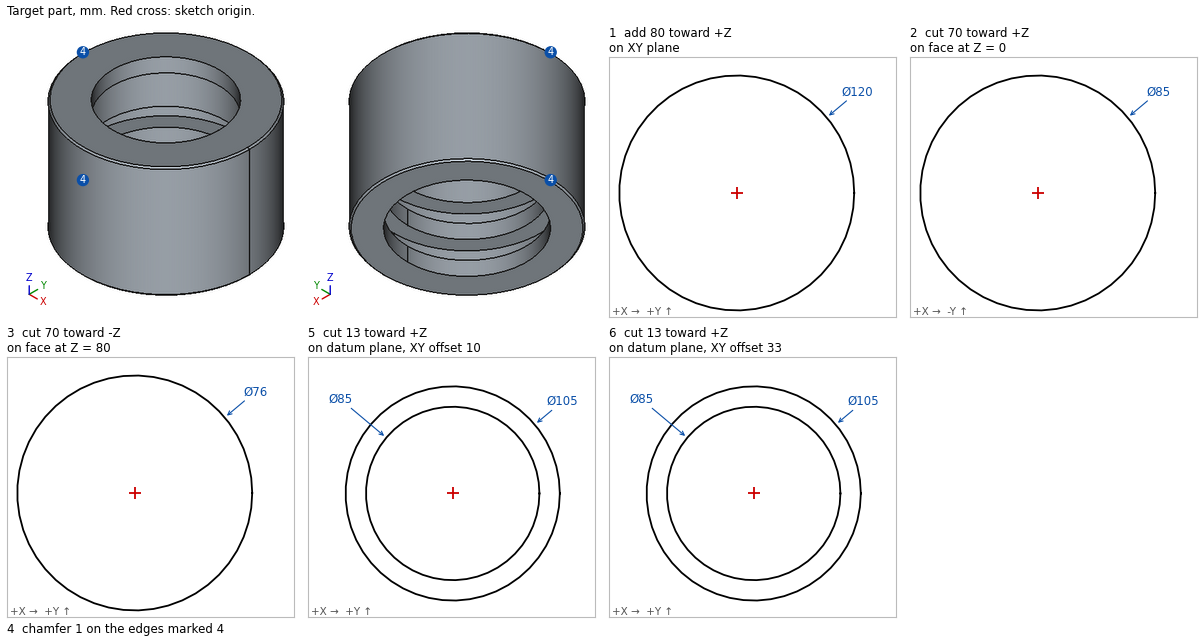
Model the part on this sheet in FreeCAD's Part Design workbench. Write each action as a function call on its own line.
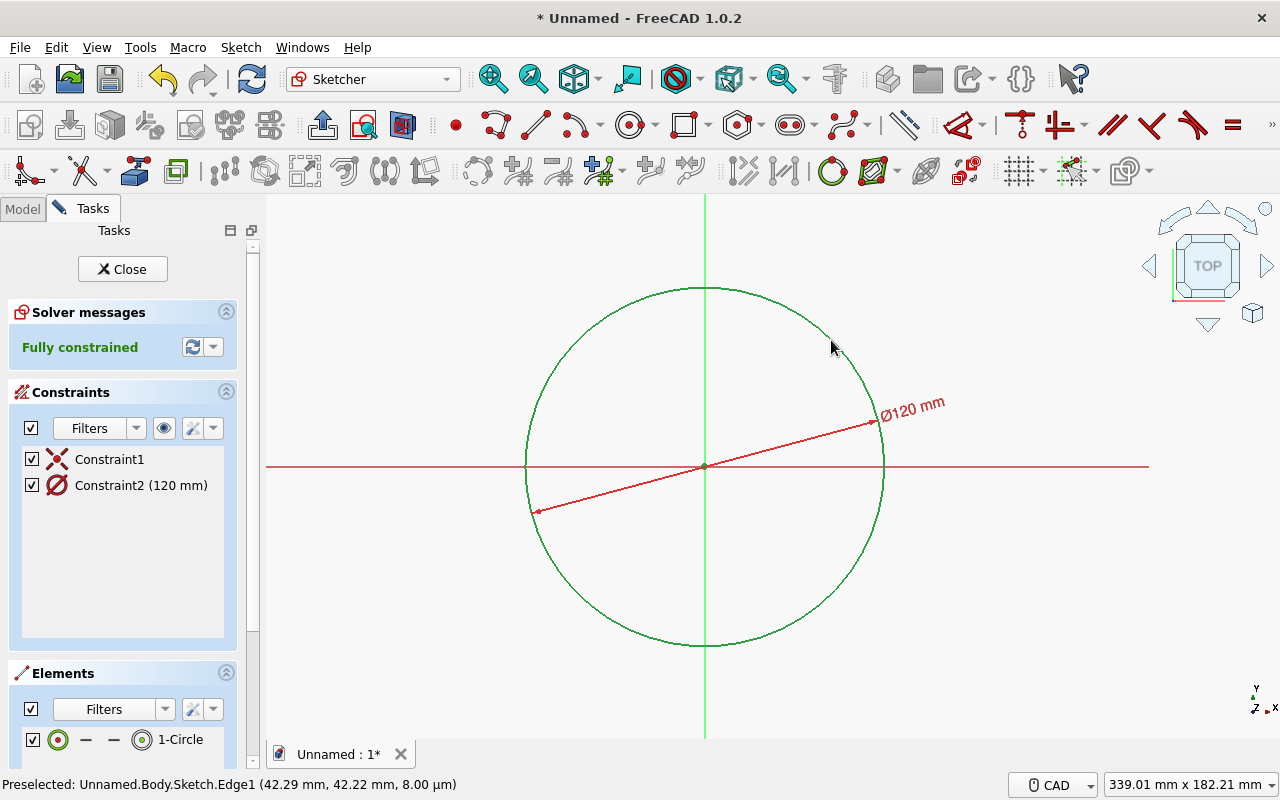
click(123, 269)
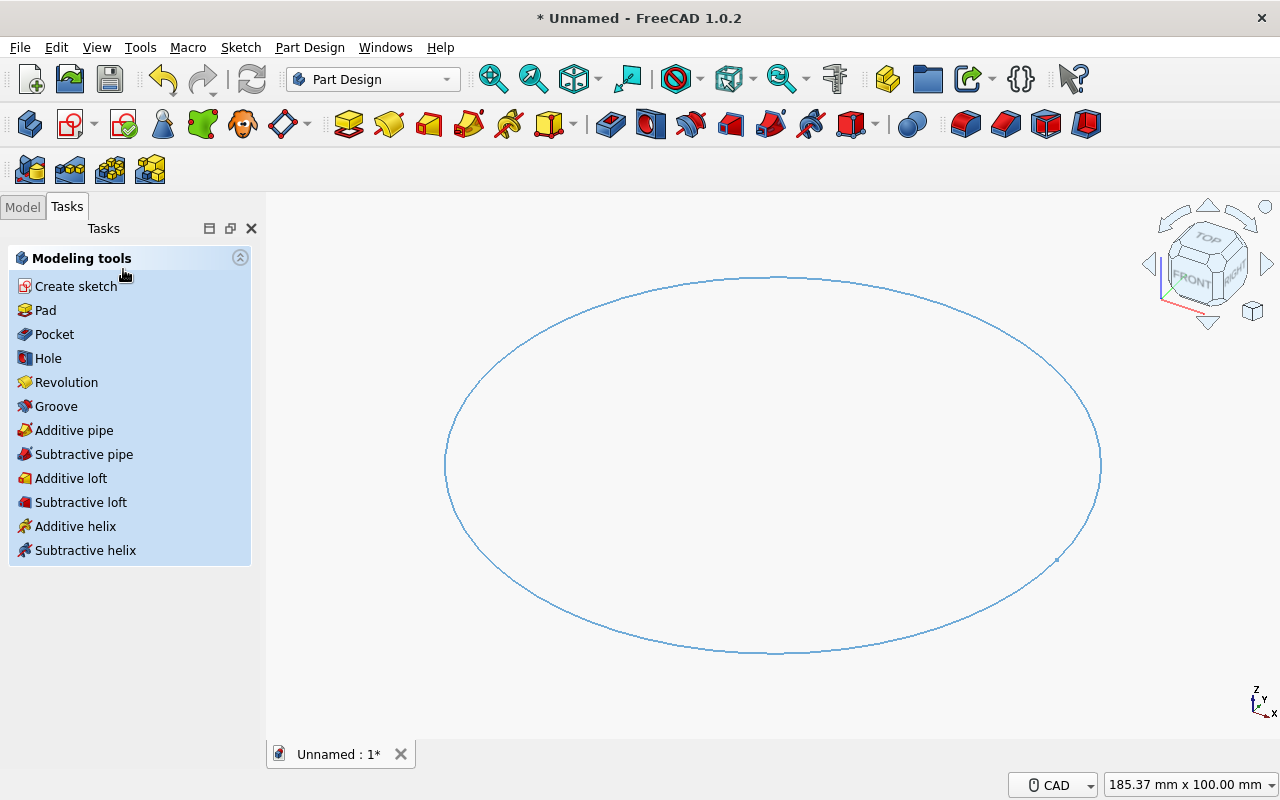
click(350, 124)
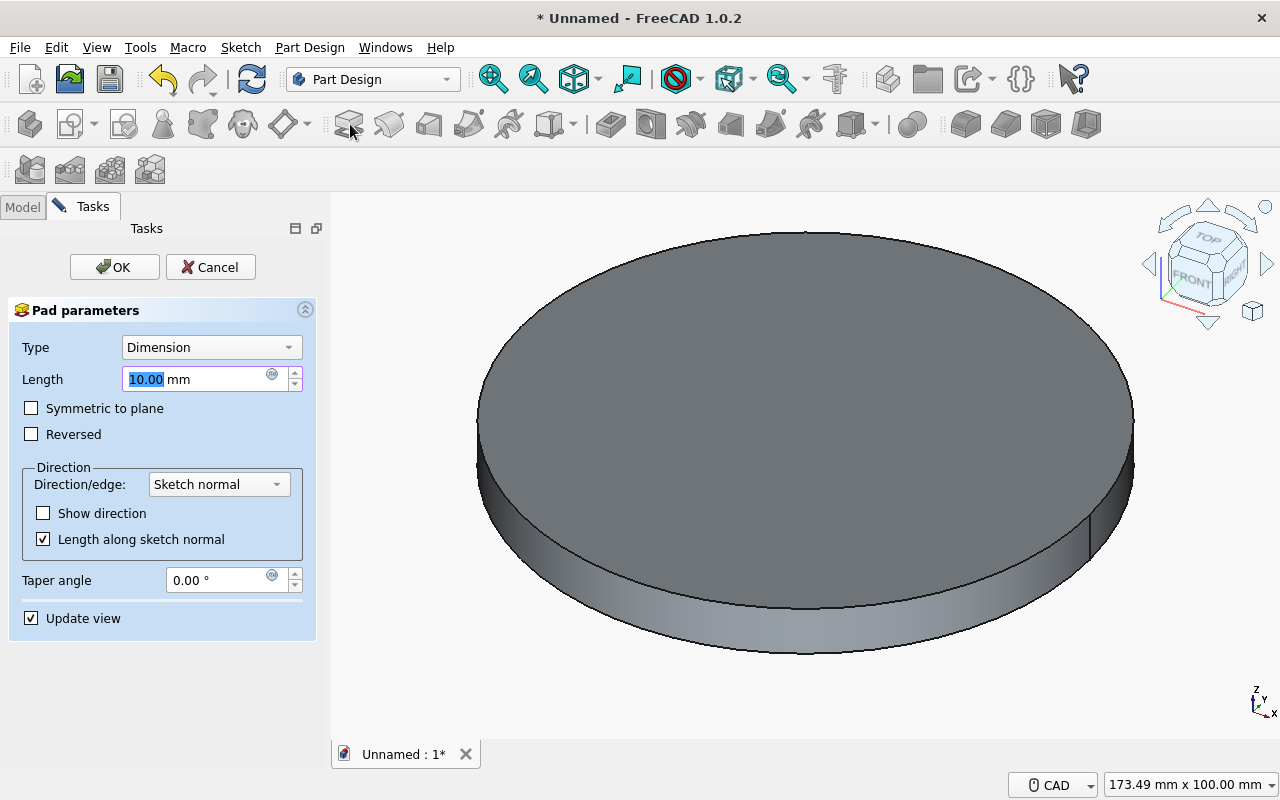
text(80)
key(Tab)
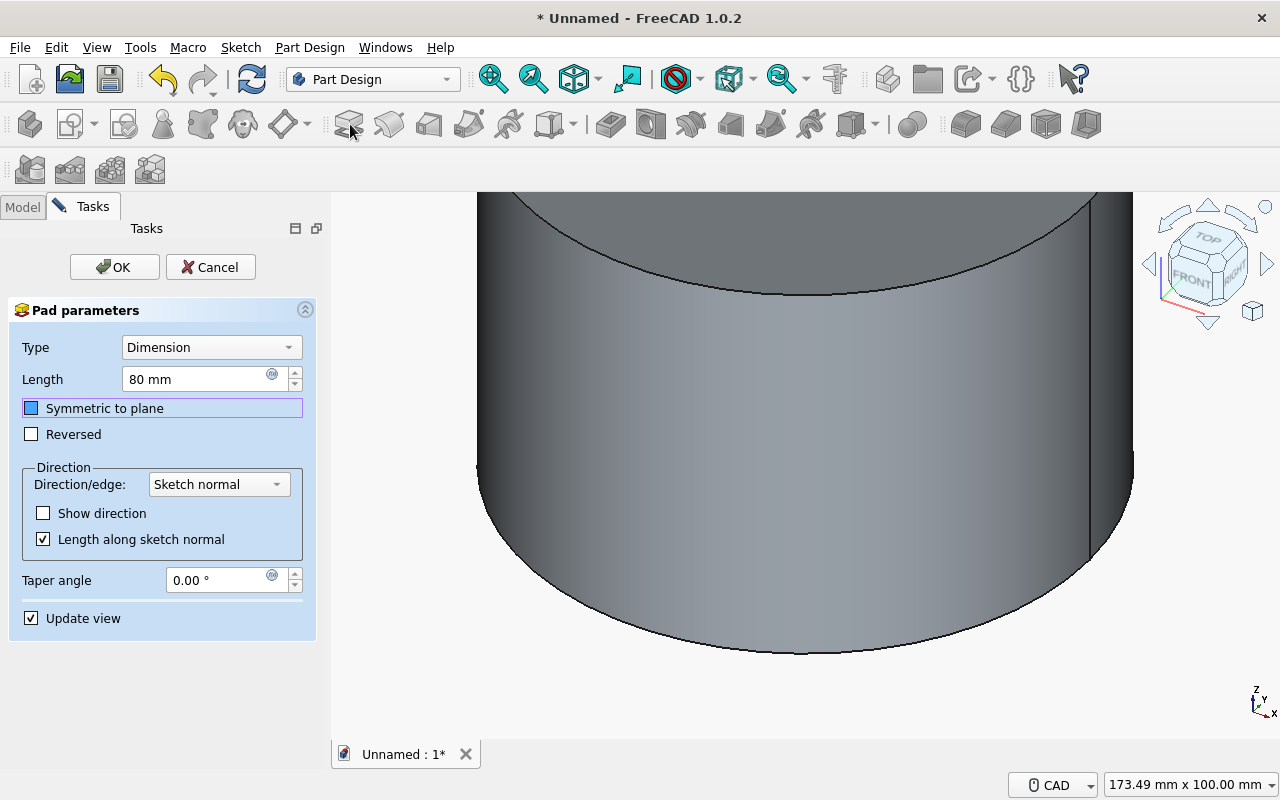
click(115, 267)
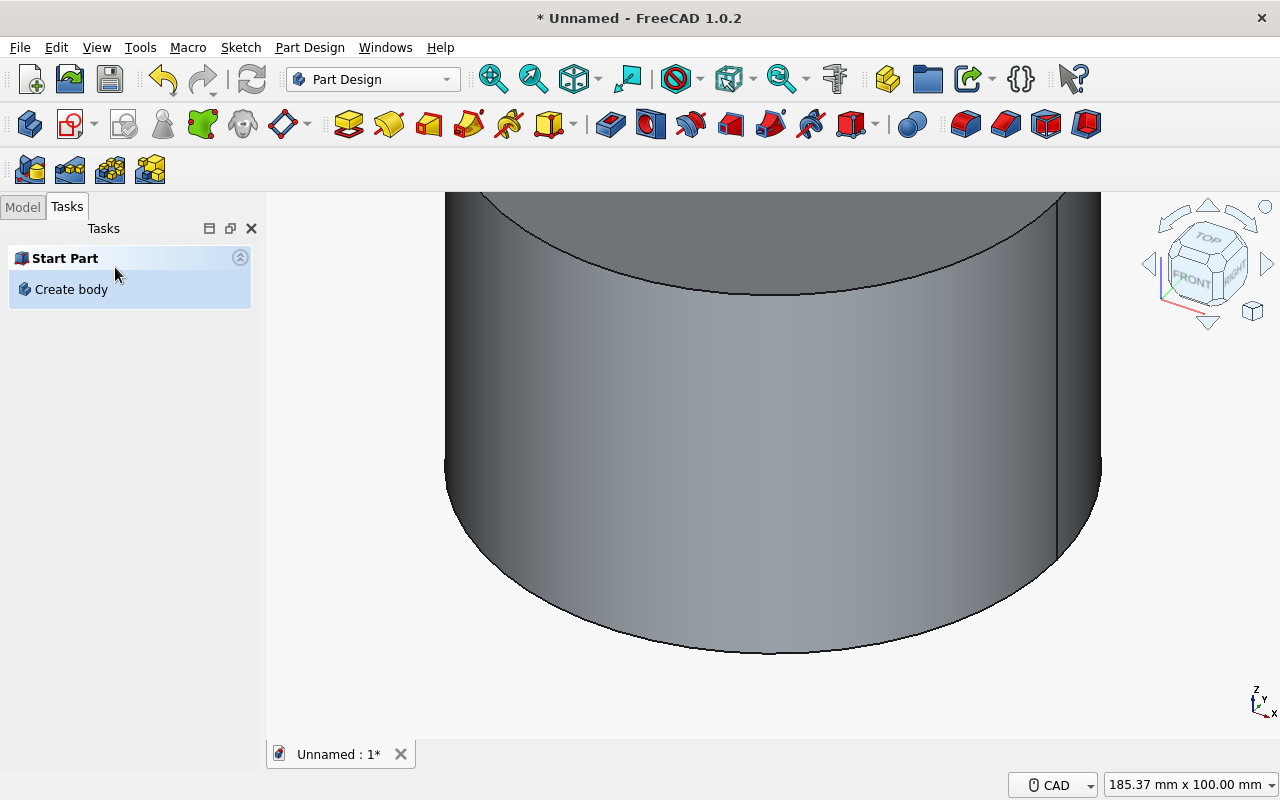
click(494, 80)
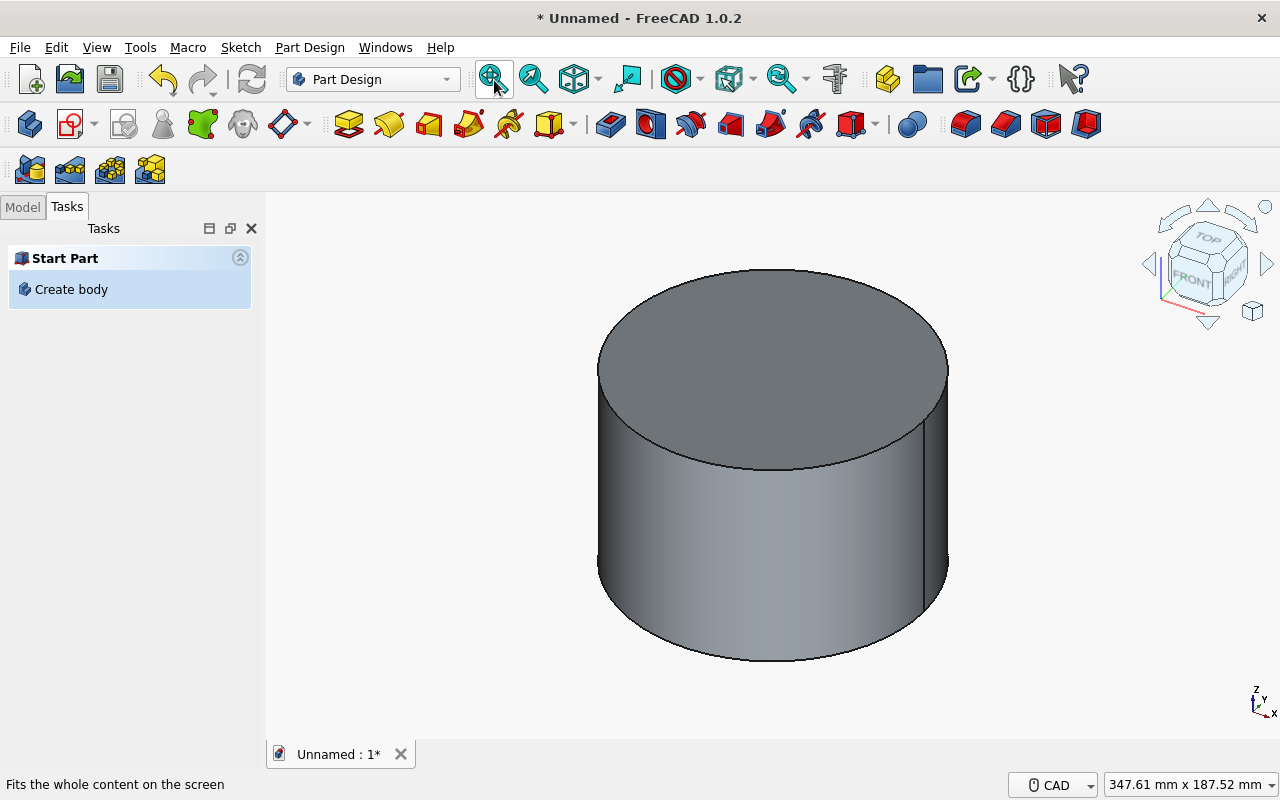
key(5)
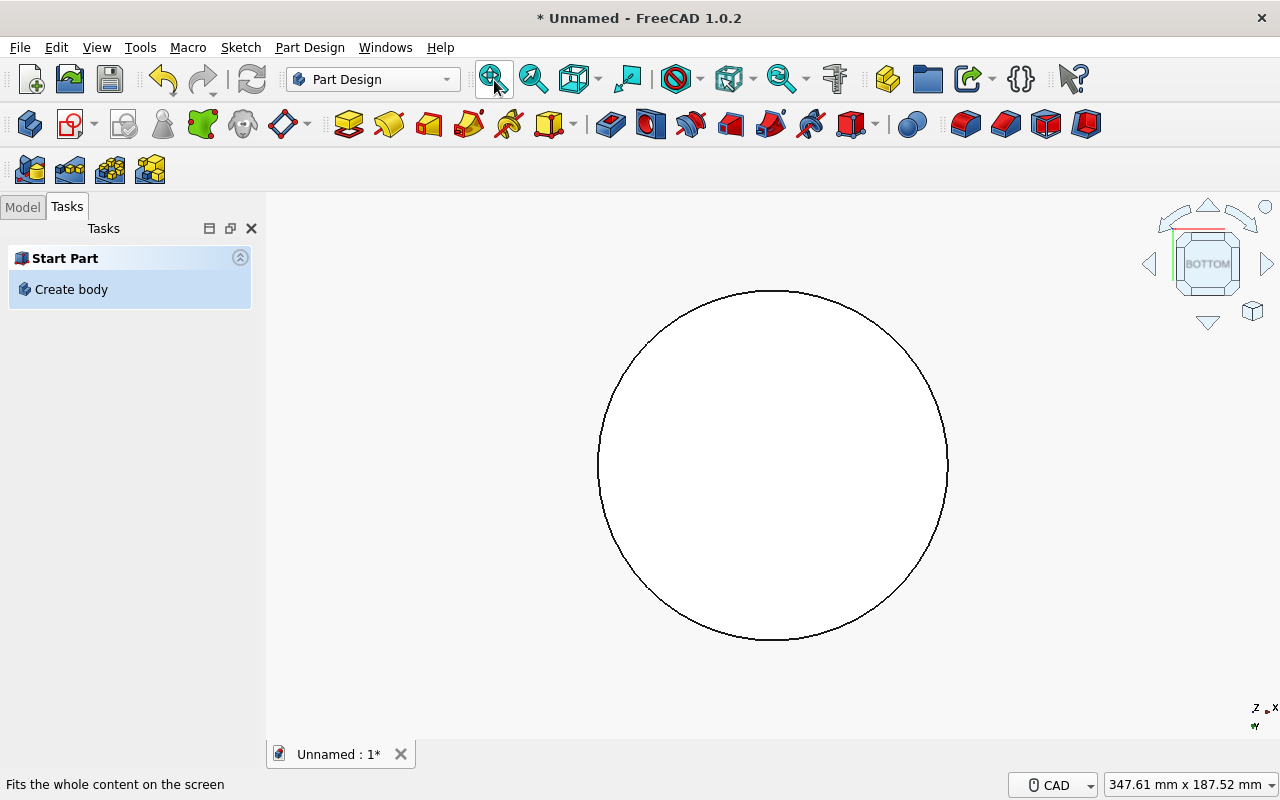
click(773, 464)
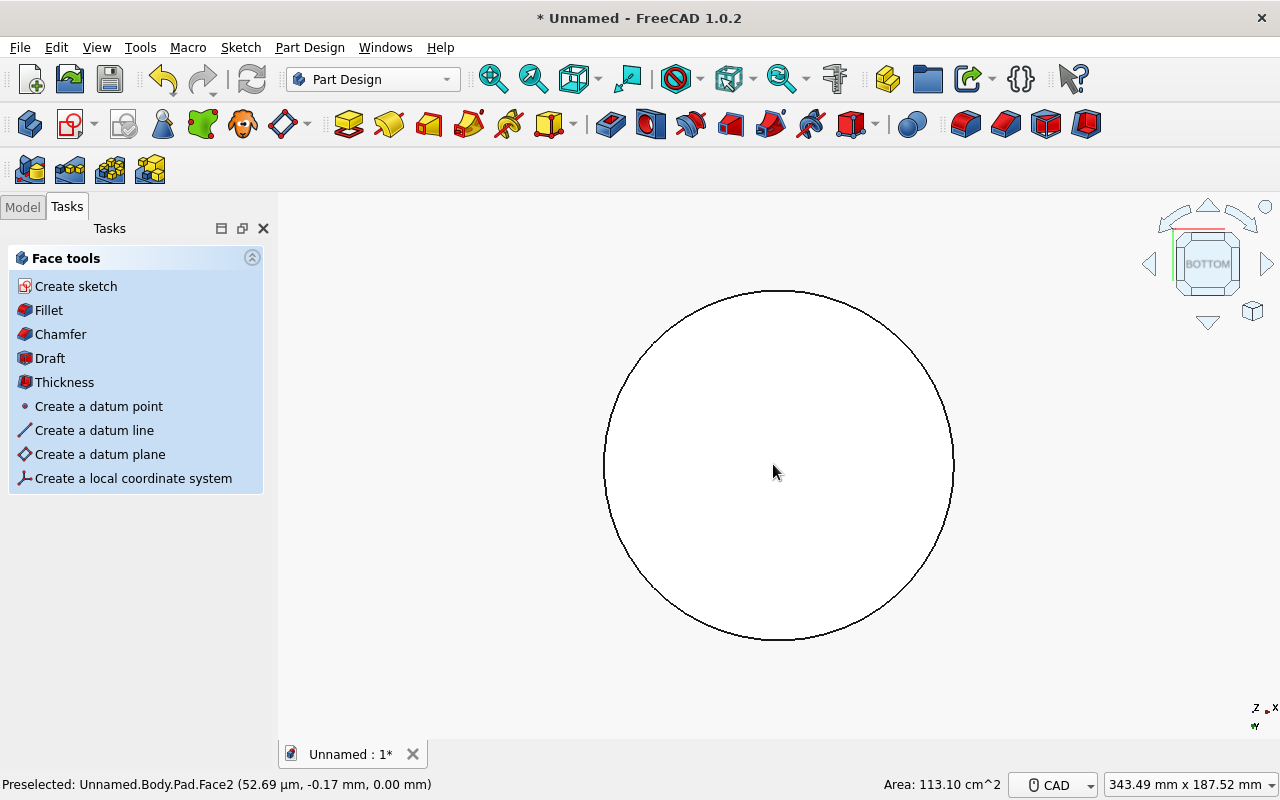
click(70, 124)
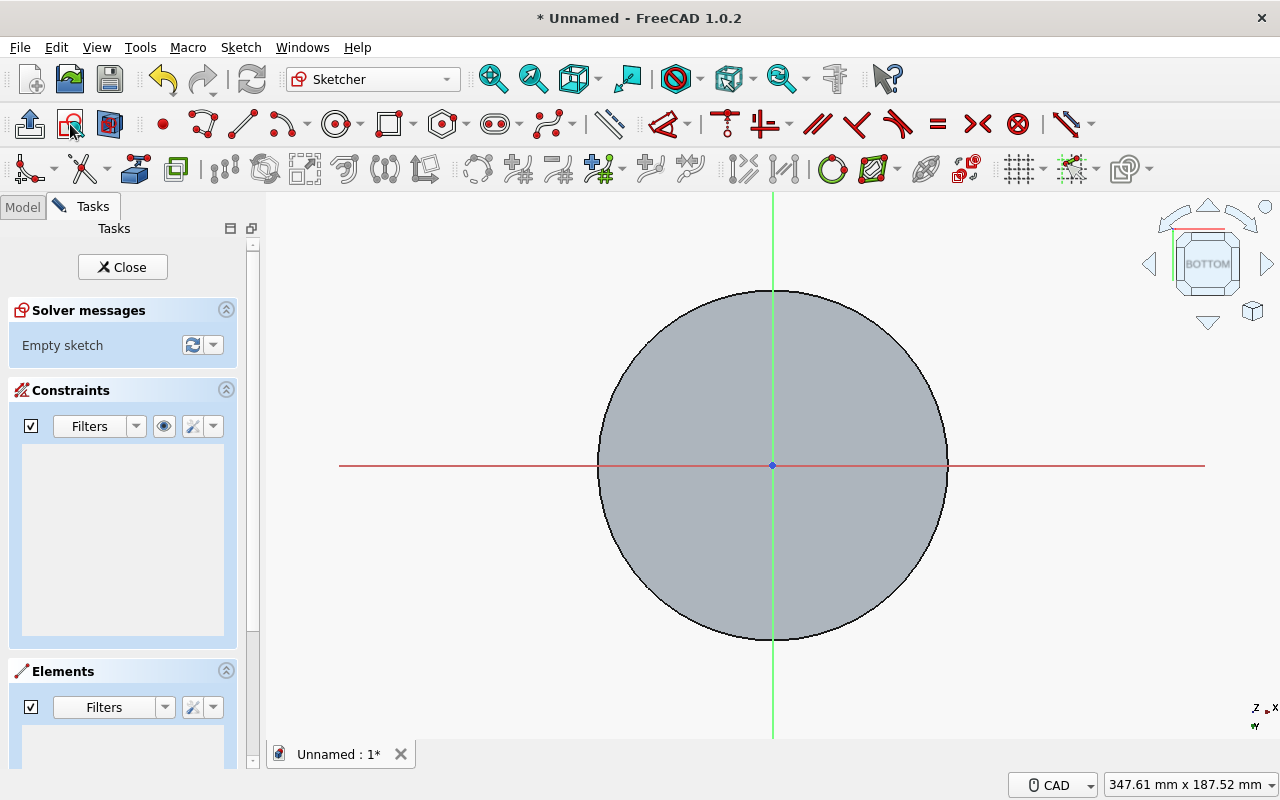
scroll(912, 466, up, 2)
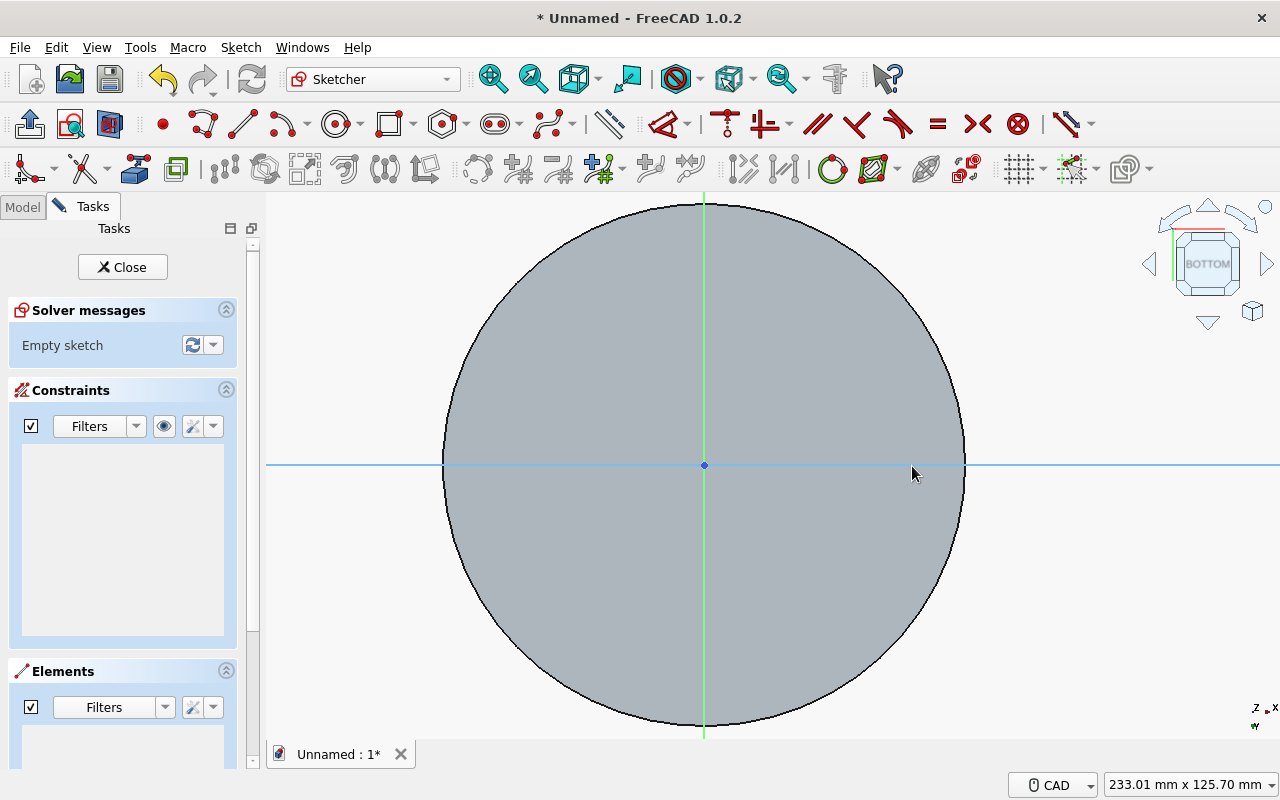
click(336, 124)